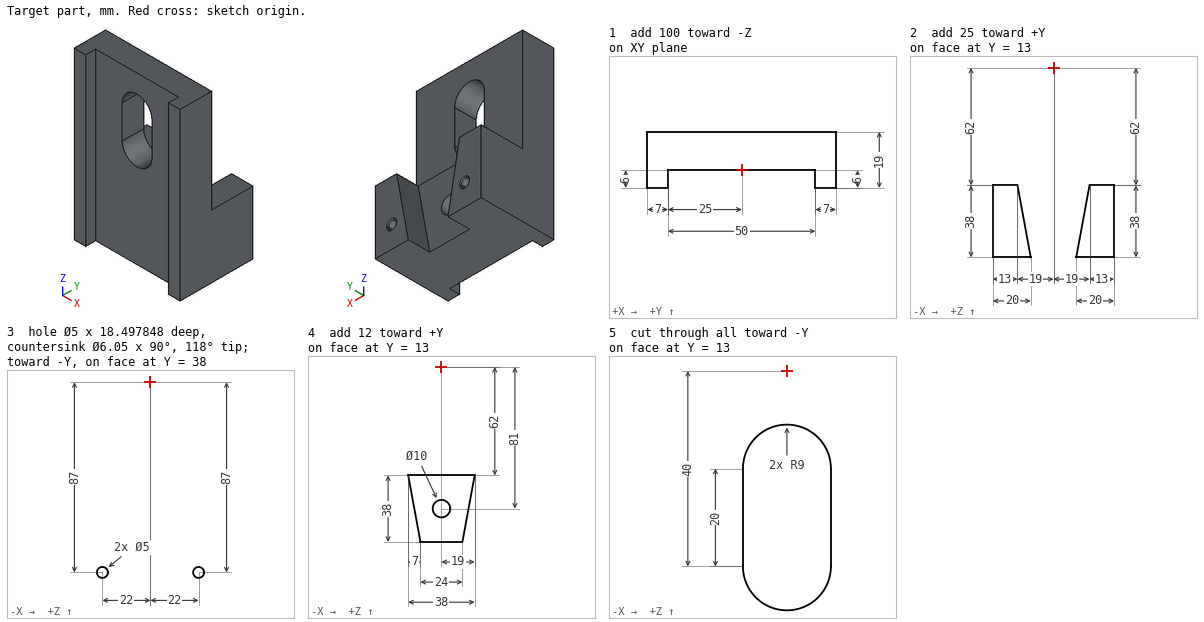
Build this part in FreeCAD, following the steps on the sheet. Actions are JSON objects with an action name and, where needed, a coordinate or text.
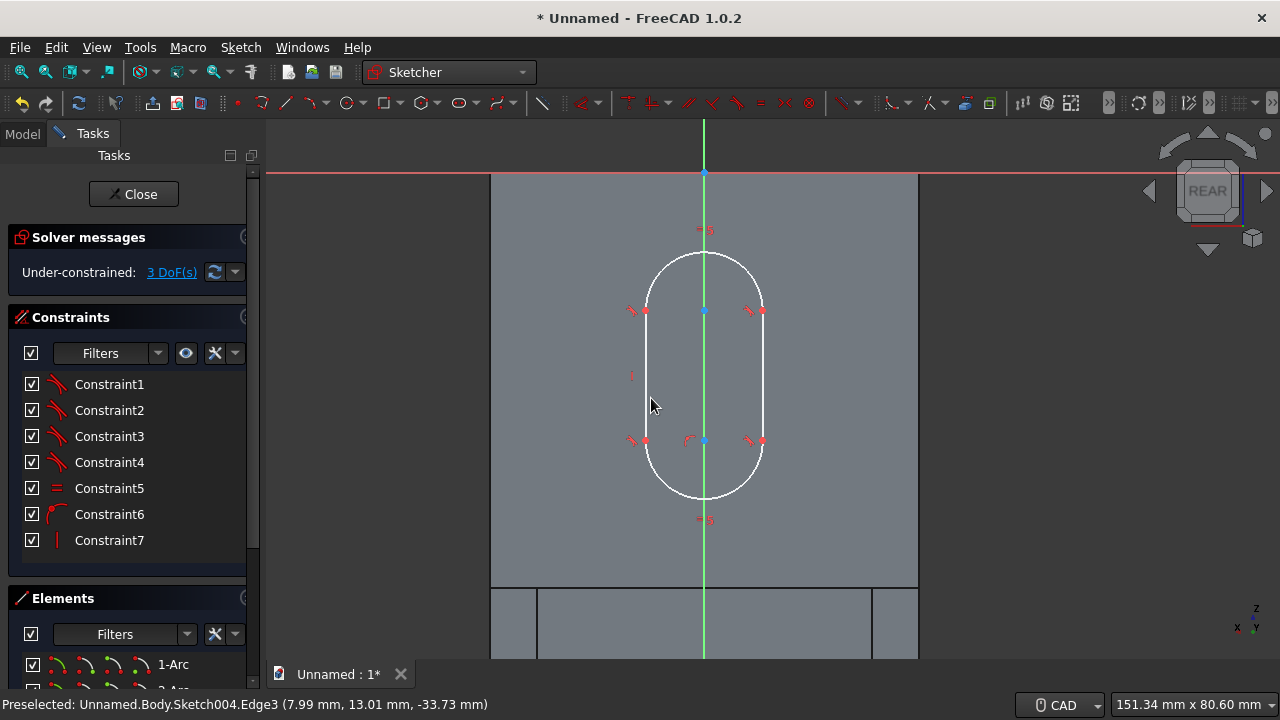
{"action": "key", "text": "d"}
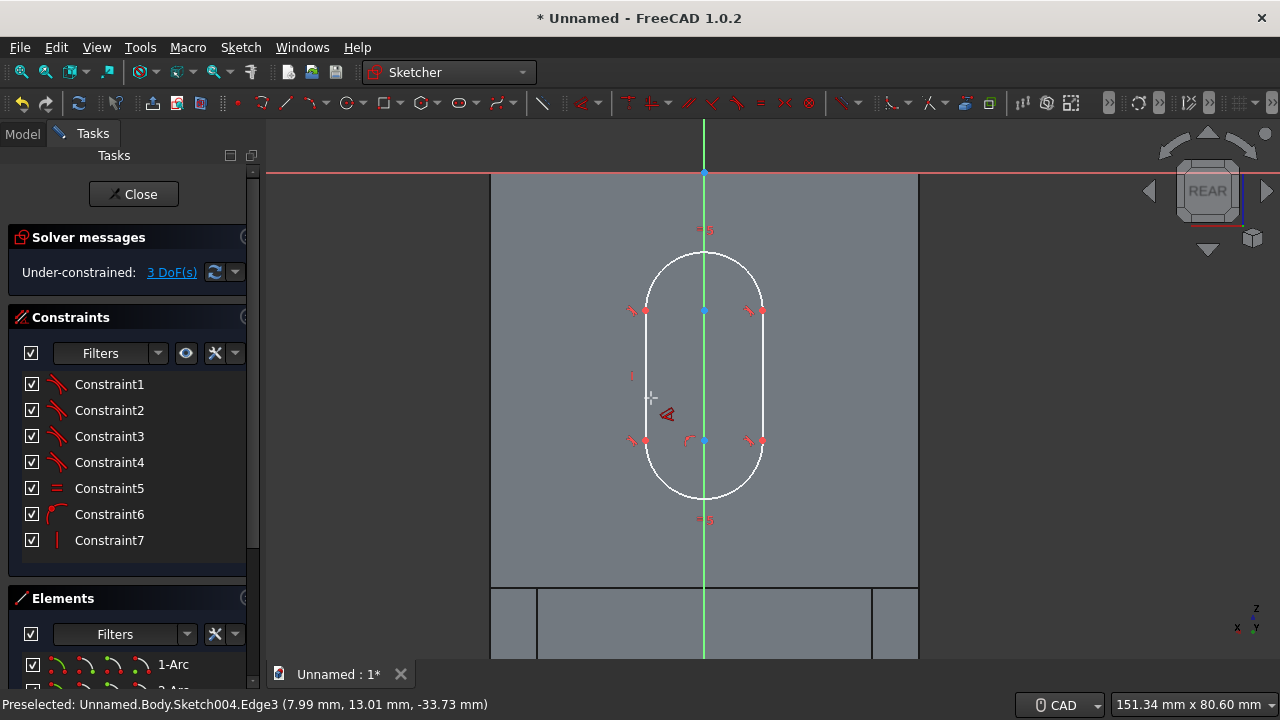
{"action": "left_click", "coordinate": [670, 488]}
{"action": "left_click", "coordinate": [651, 514]}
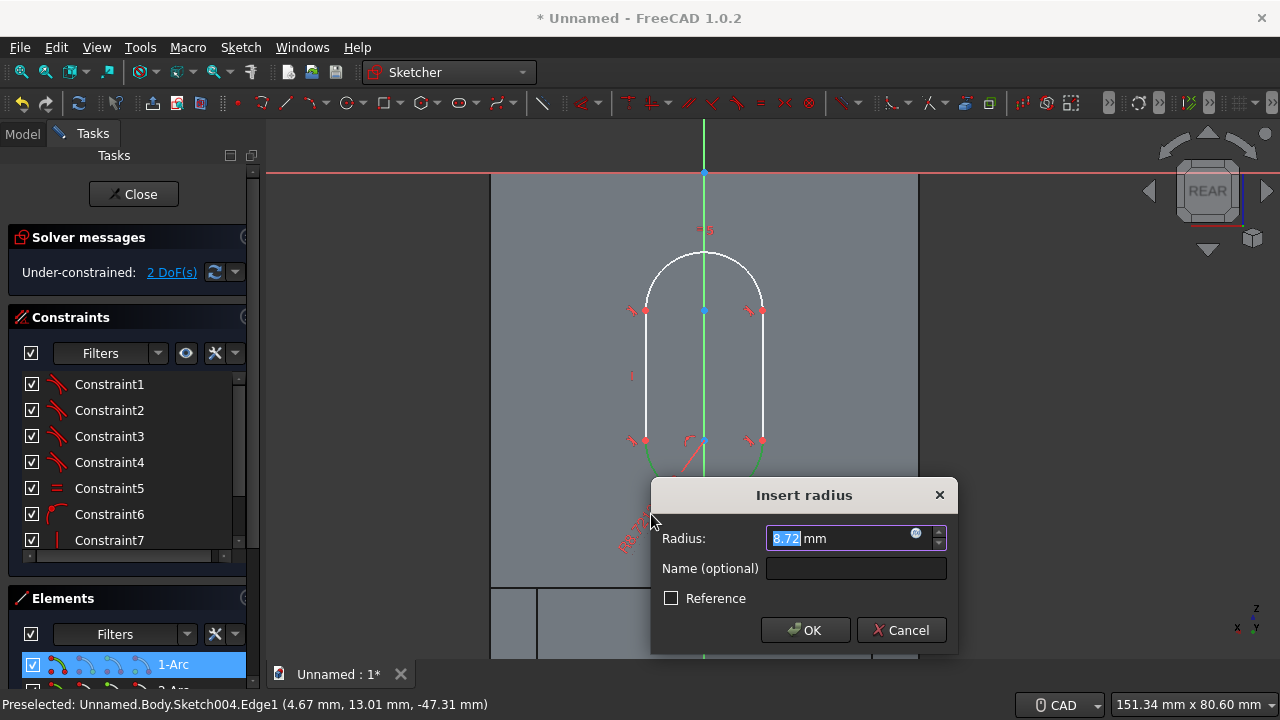
{"action": "type", "text": "9"}
{"action": "key", "text": "Return"}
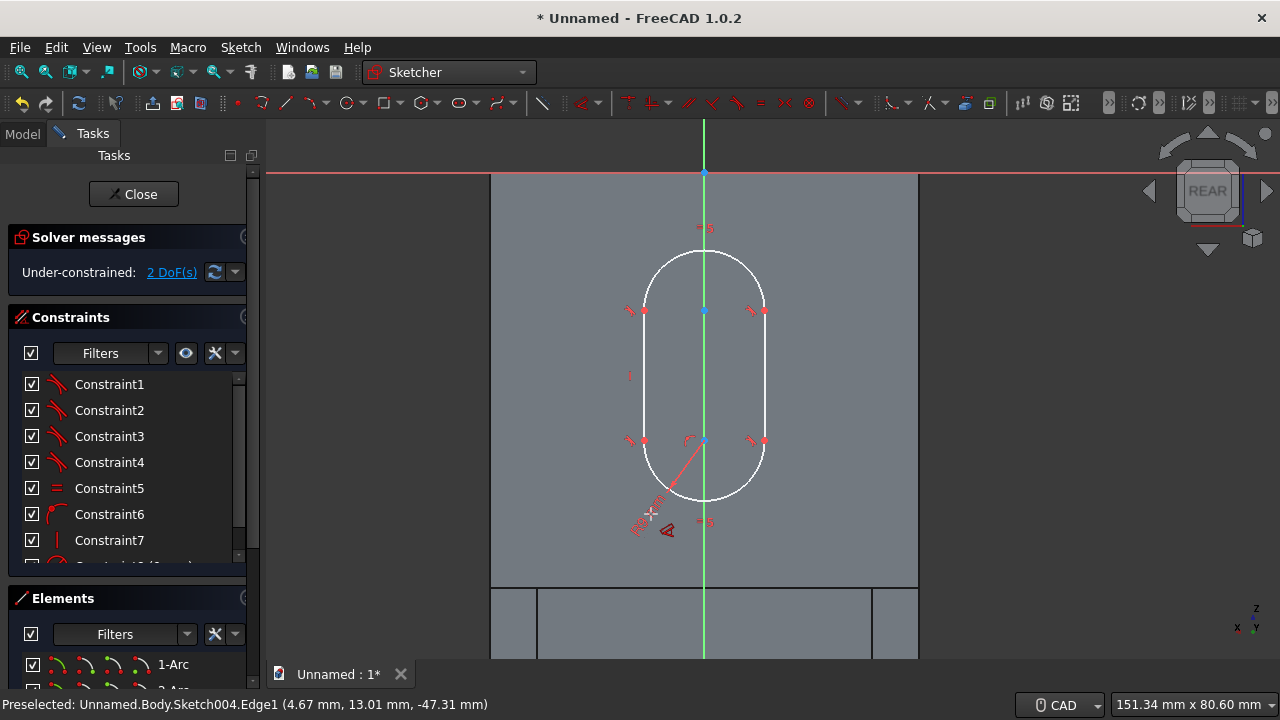
{"action": "left_click", "coordinate": [644, 402]}
{"action": "left_click", "coordinate": [610, 376]}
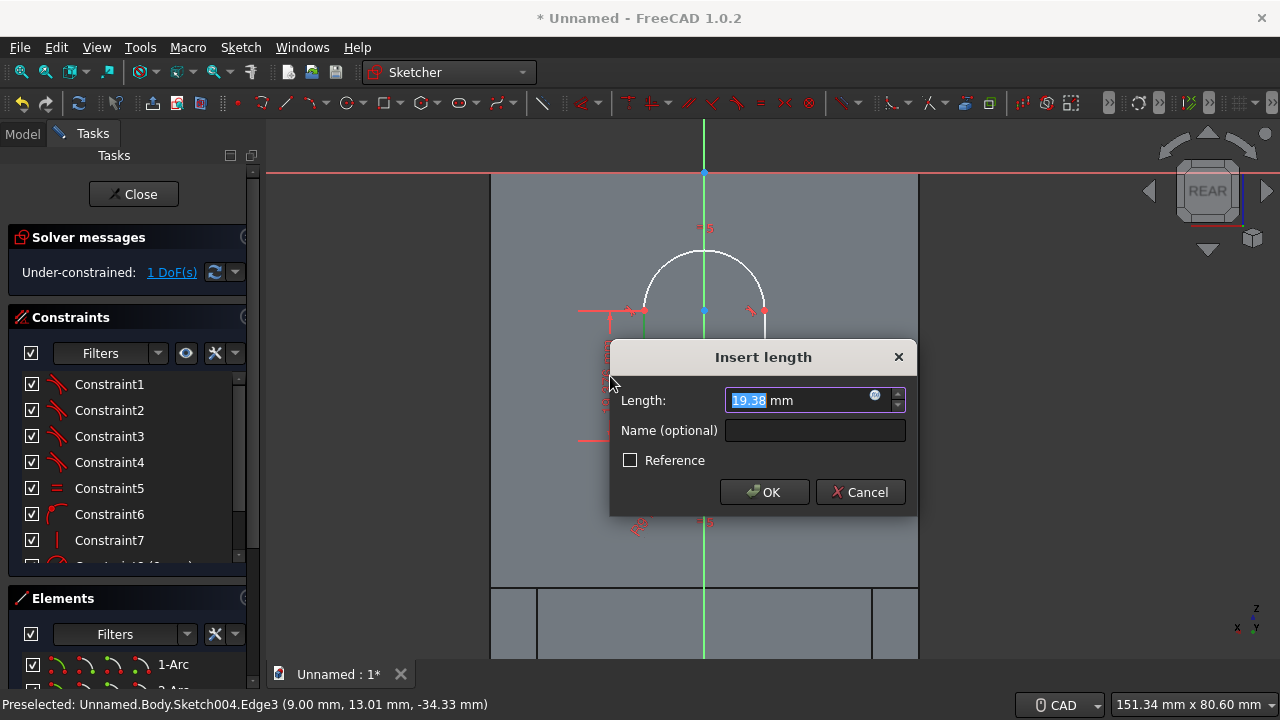
{"action": "type", "text": "20"}
{"action": "key", "text": "Return"}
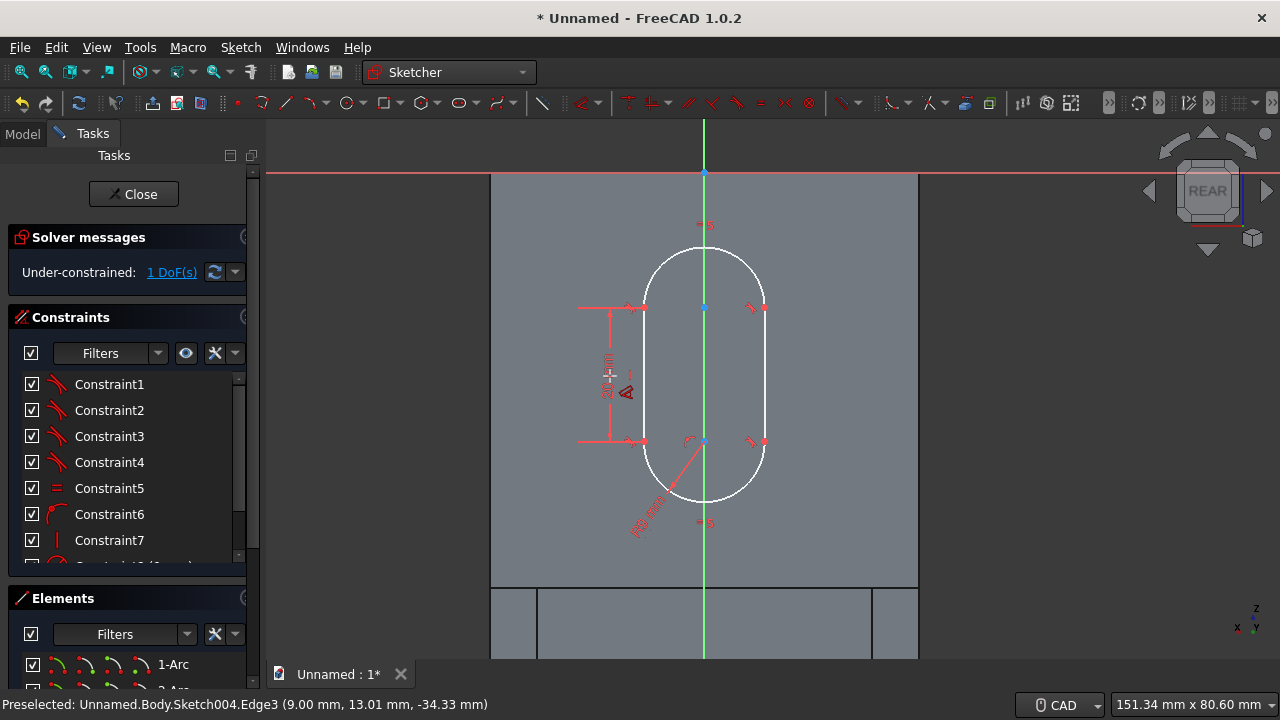
{"action": "left_click", "coordinate": [644, 442]}
{"action": "left_click", "coordinate": [610, 307]}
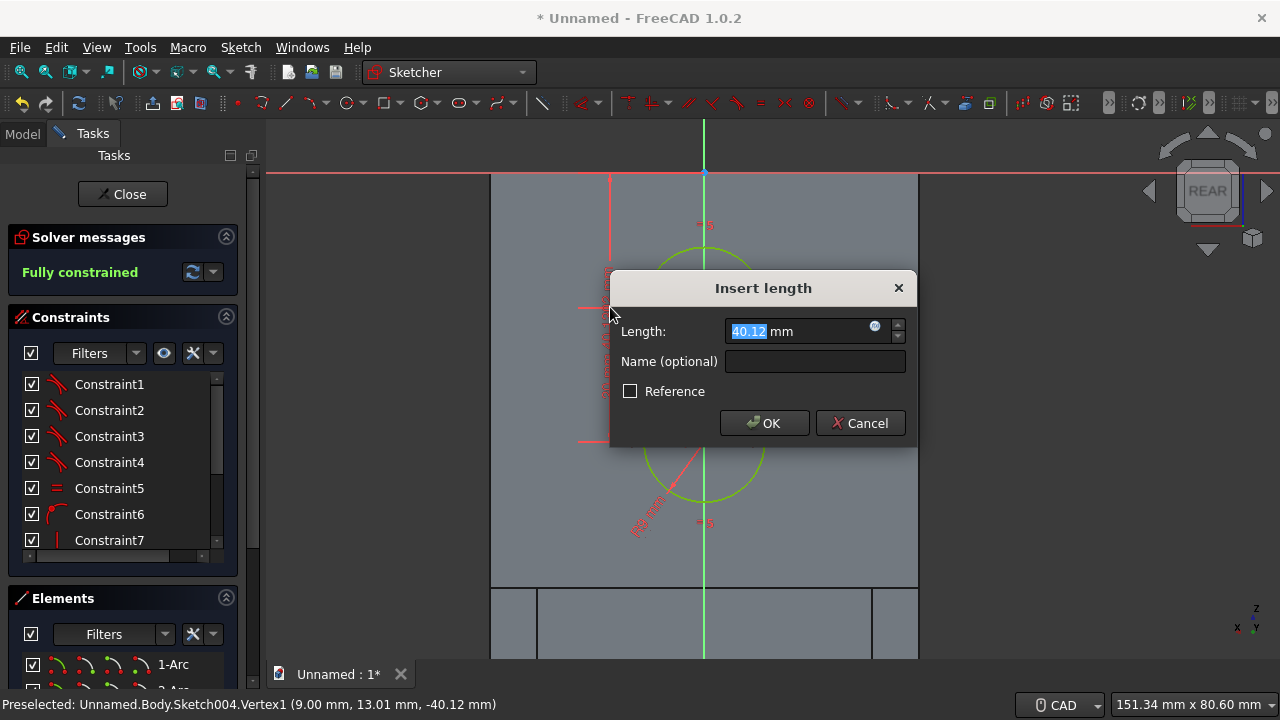
{"action": "type", "text": "40"}
{"action": "key", "text": "Return"}
{"action": "key", "text": "Escape"}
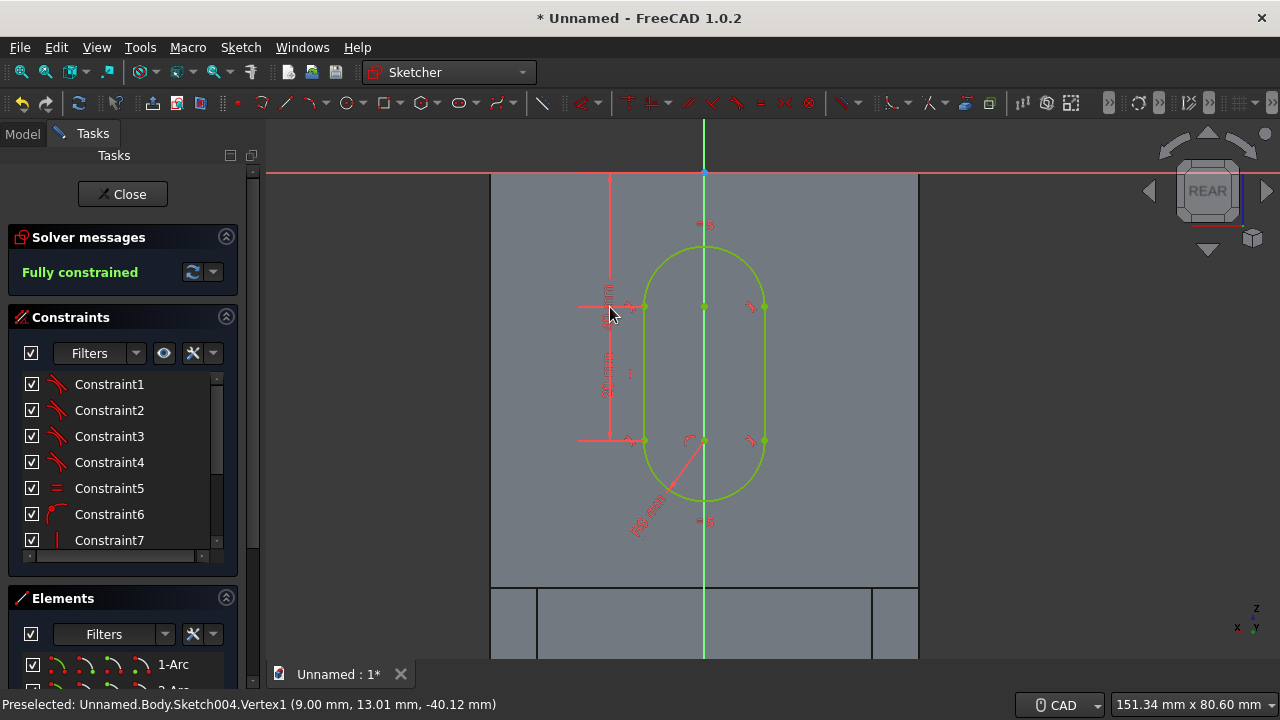
{"action": "left_click", "coordinate": [123, 194]}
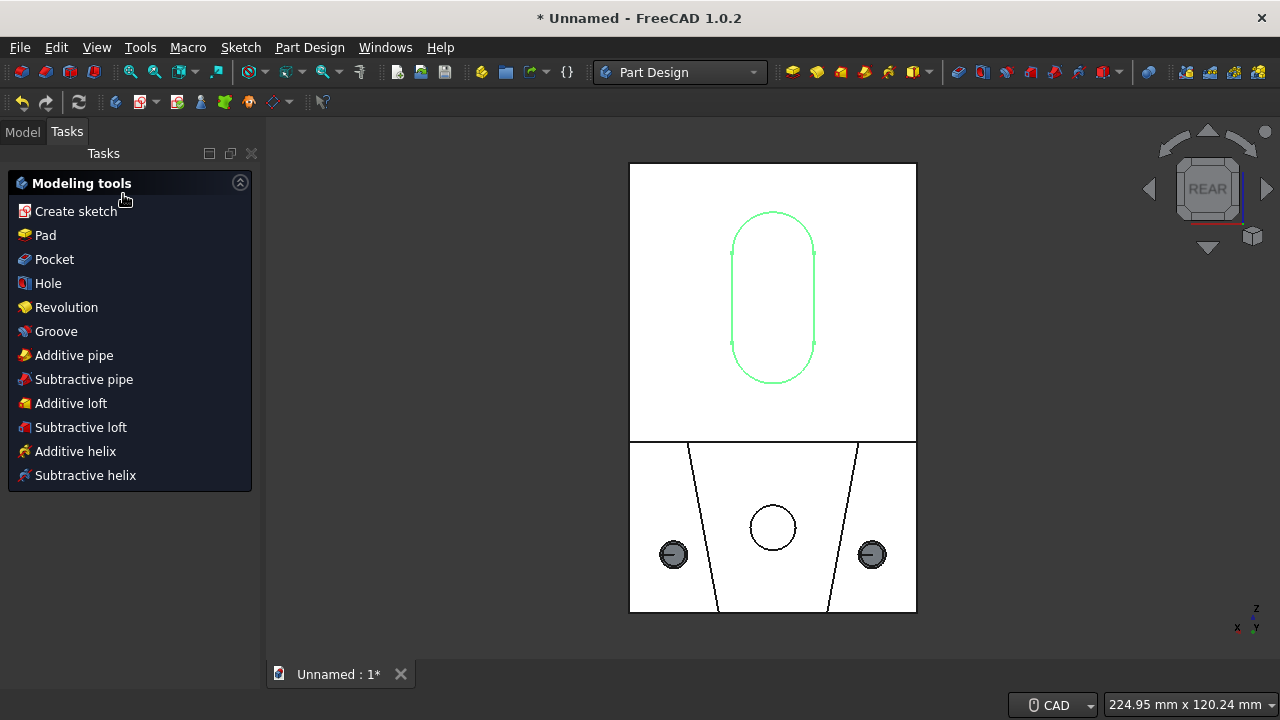
{"action": "left_click", "coordinate": [960, 72]}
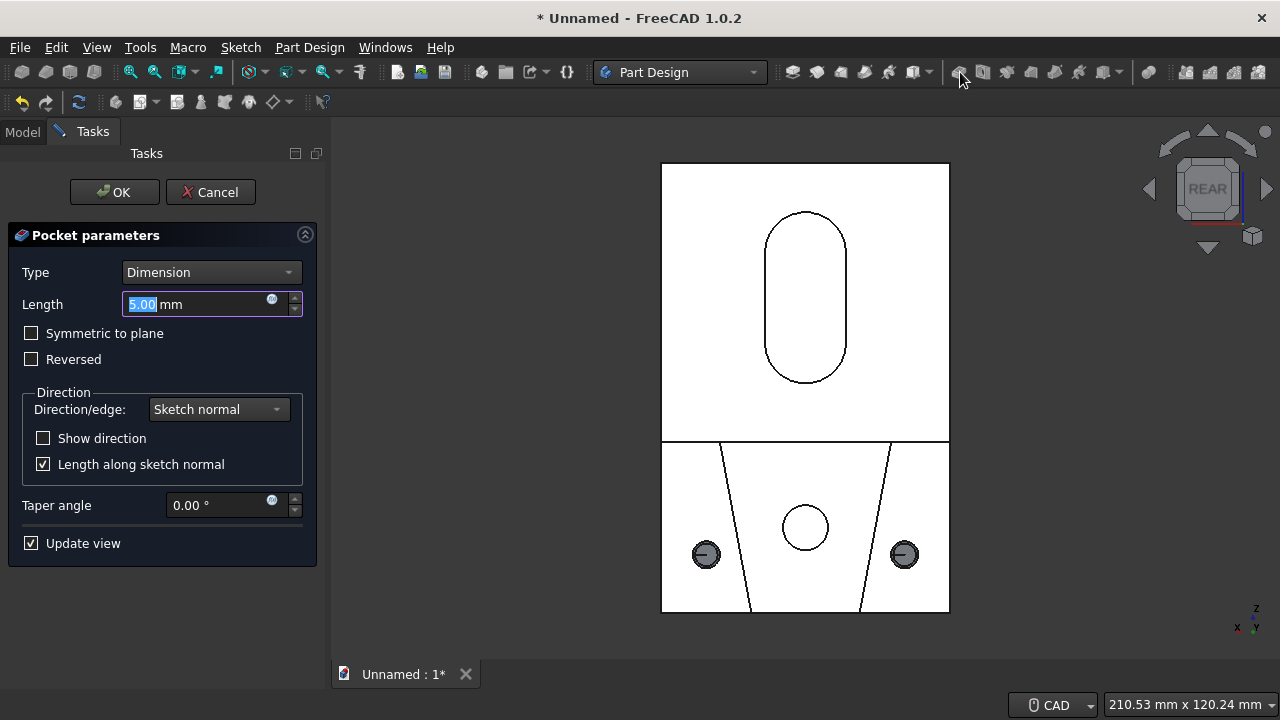
{"action": "left_click", "coordinate": [212, 272]}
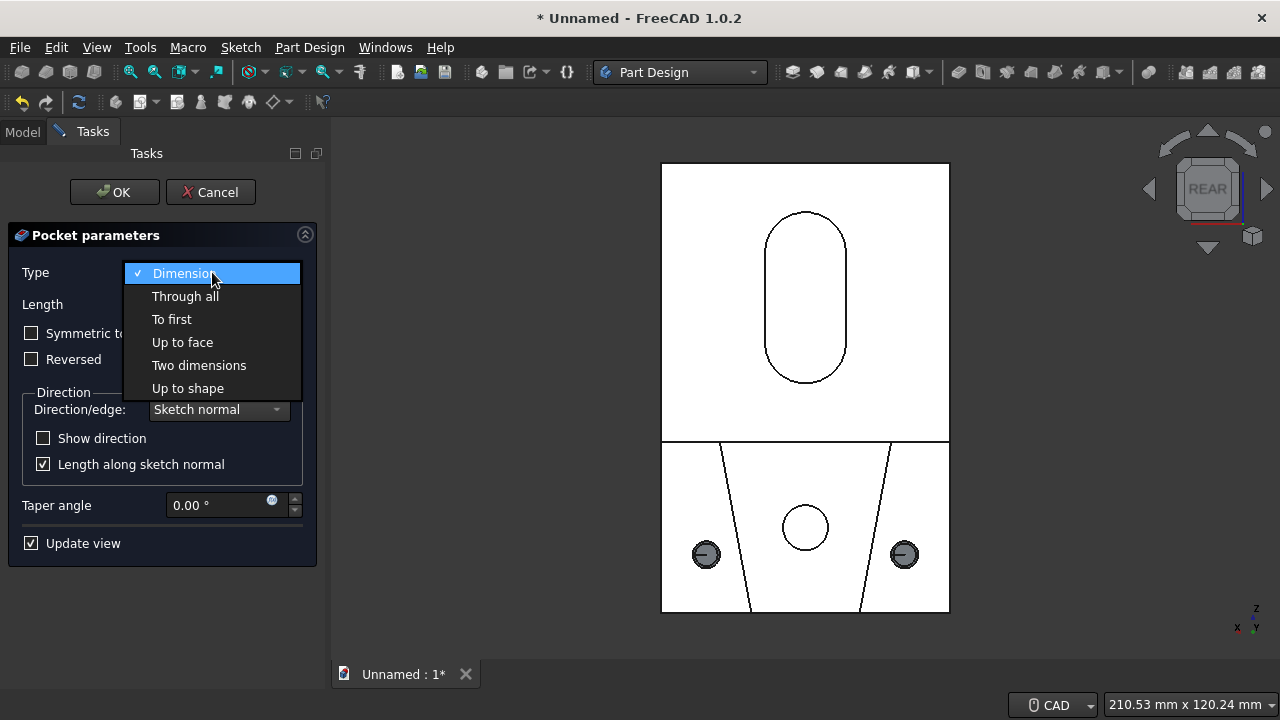
{"action": "left_click", "coordinate": [212, 296]}